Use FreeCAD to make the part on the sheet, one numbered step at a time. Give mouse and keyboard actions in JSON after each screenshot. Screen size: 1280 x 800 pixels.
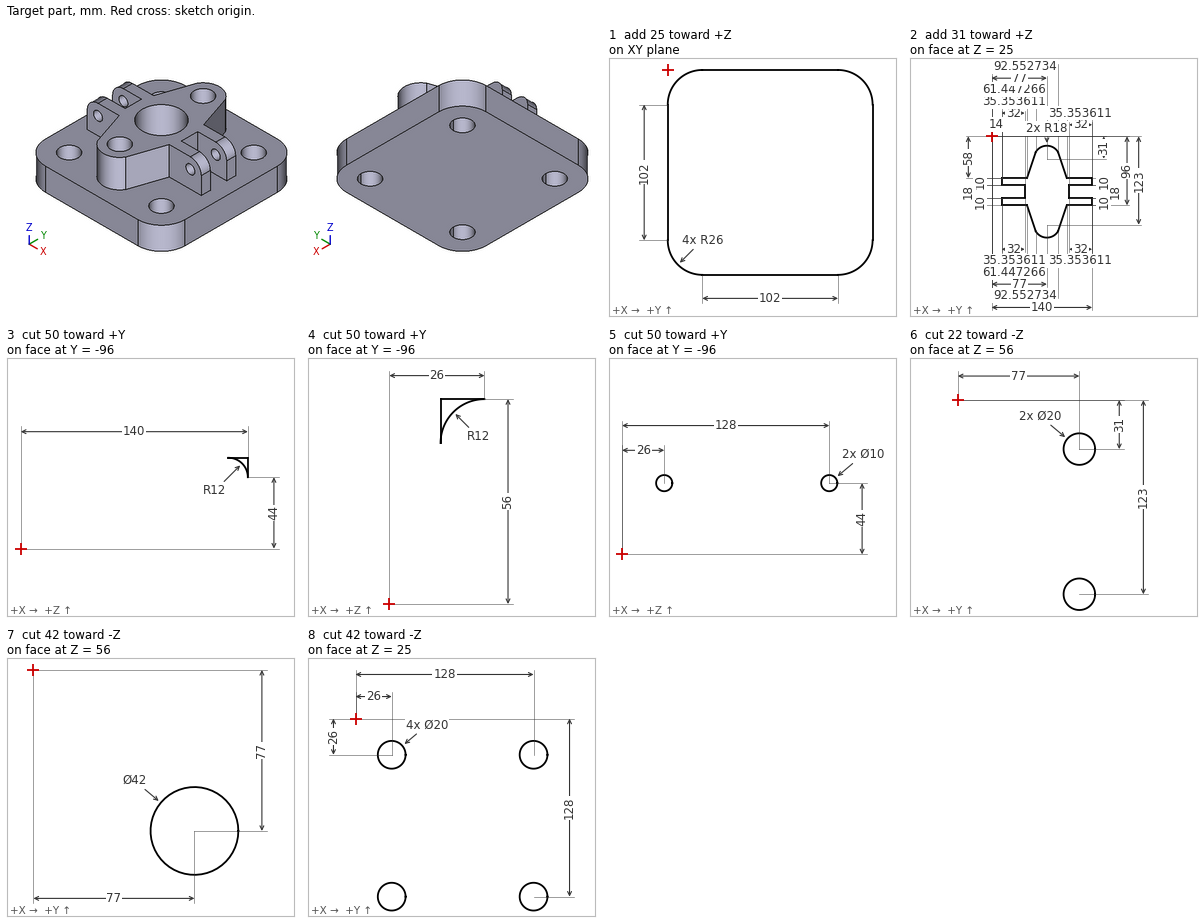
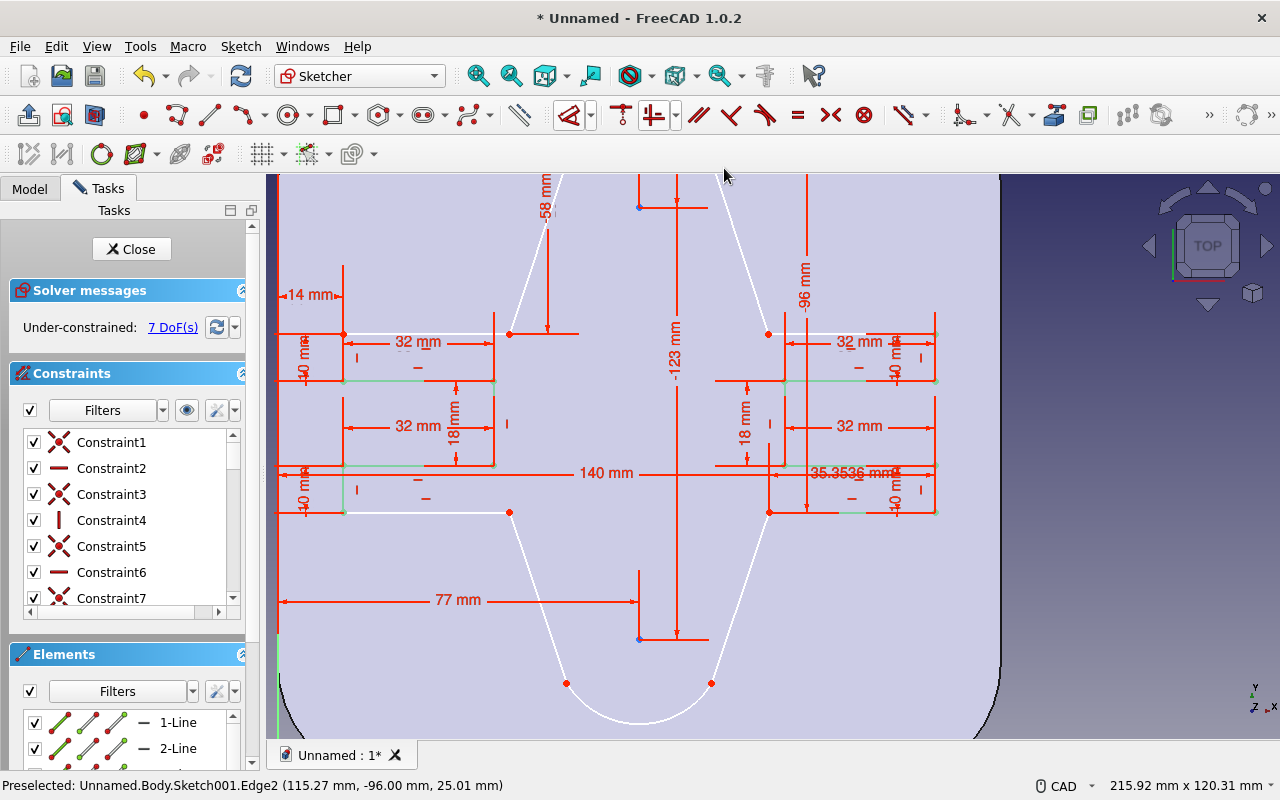
{"action": "left_click", "coordinate": [885, 334]}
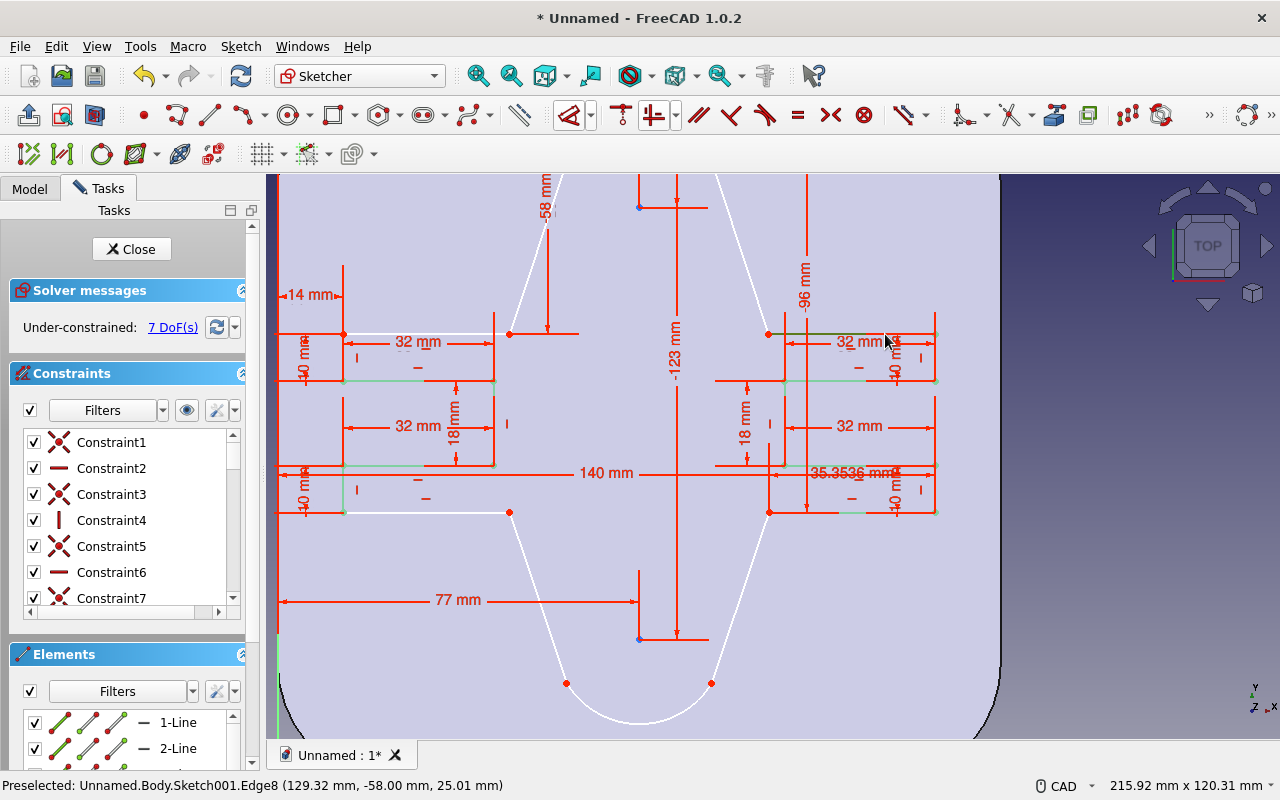
{"action": "key", "text": "l"}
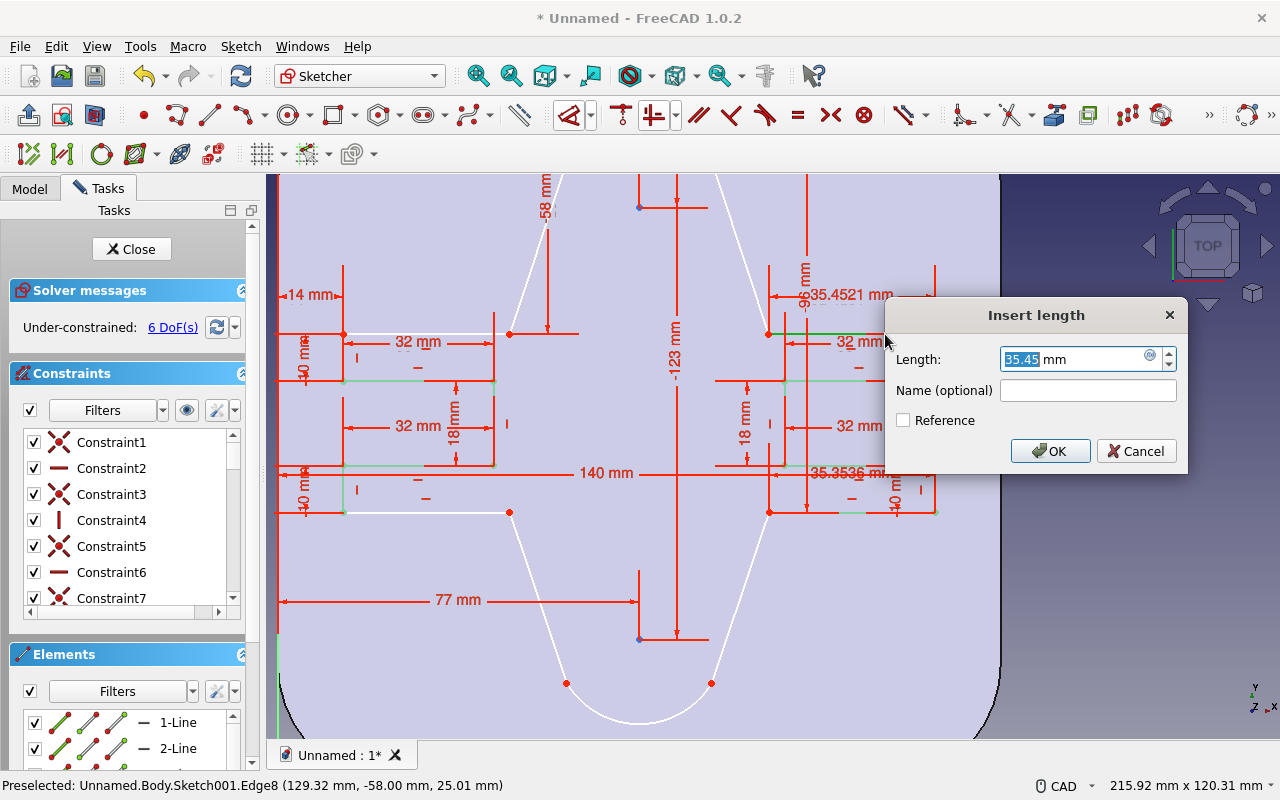
{"action": "type", "text": "35.353611"}
{"action": "key", "text": "Return"}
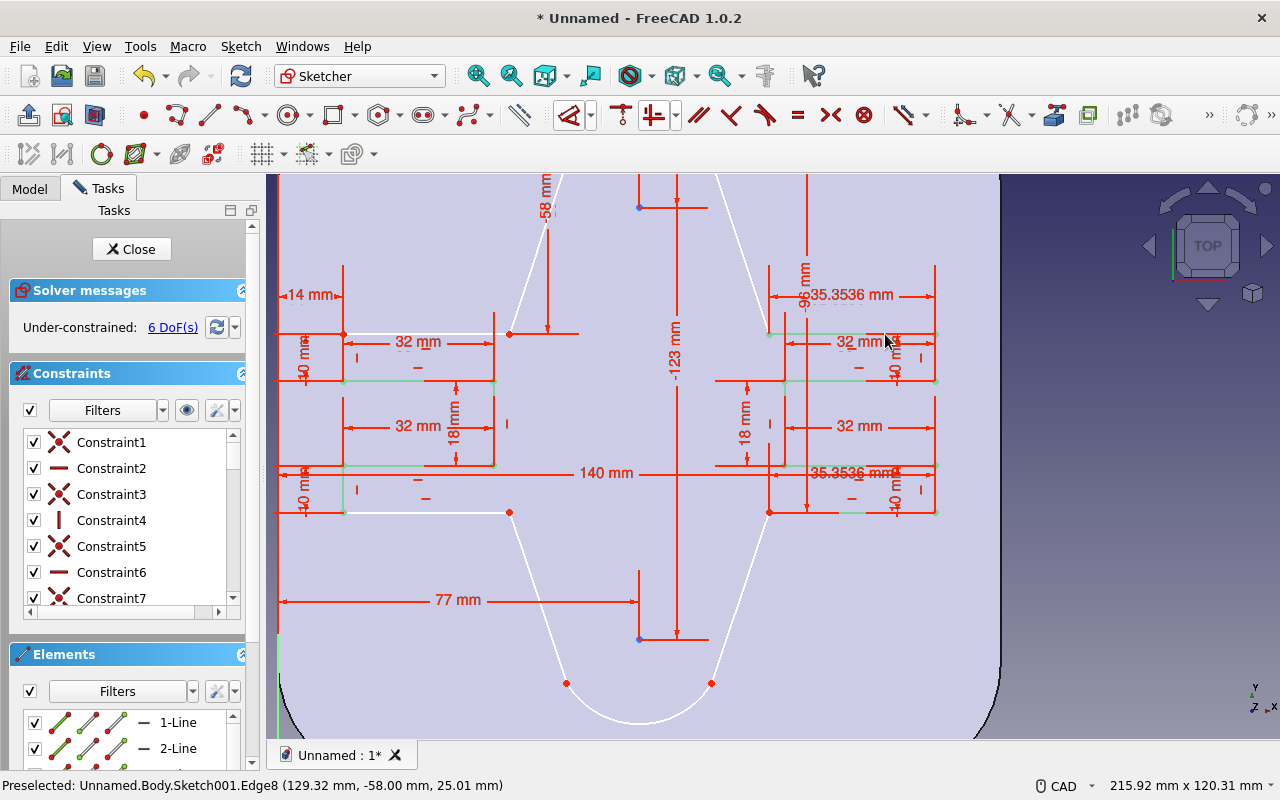
{"action": "left_click", "coordinate": [460, 334]}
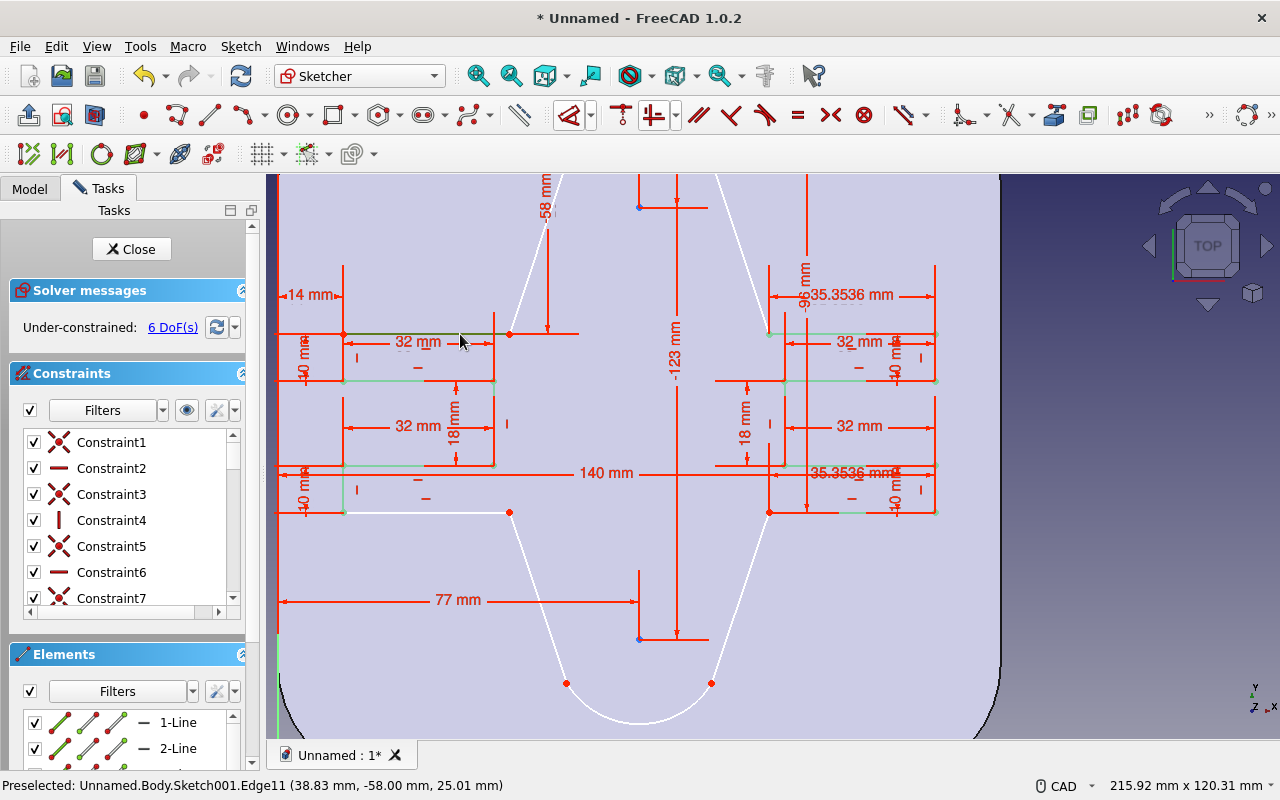
{"action": "key", "text": "l"}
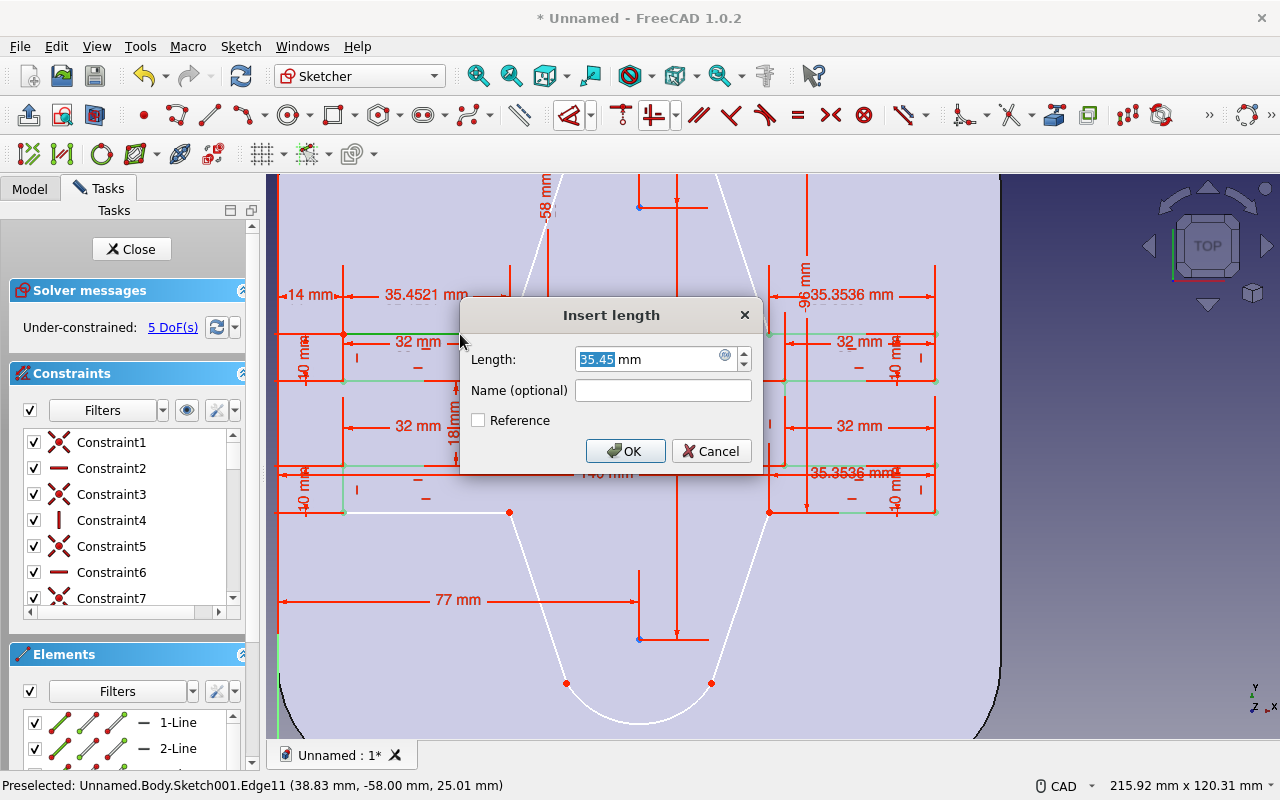
{"action": "type", "text": "35.353611"}
{"action": "key", "text": "Return"}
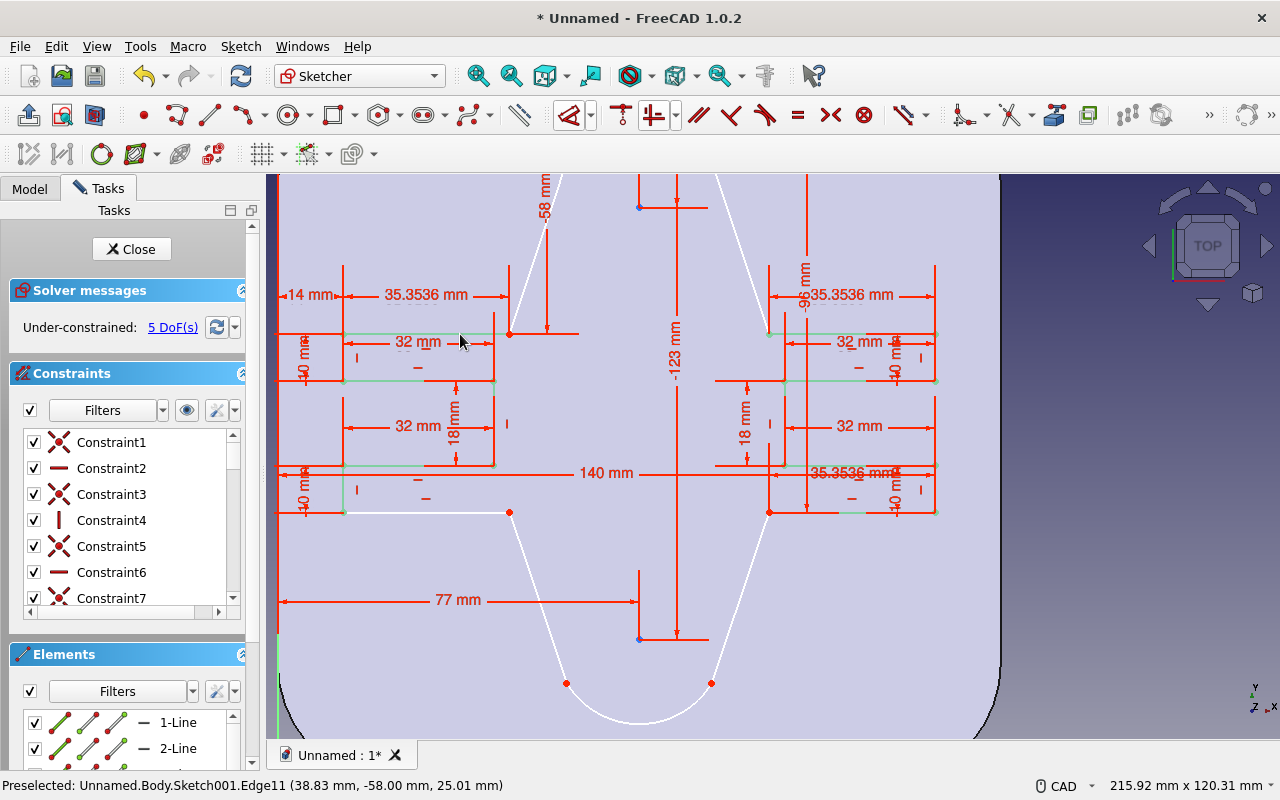
{"action": "left_click", "coordinate": [393, 513]}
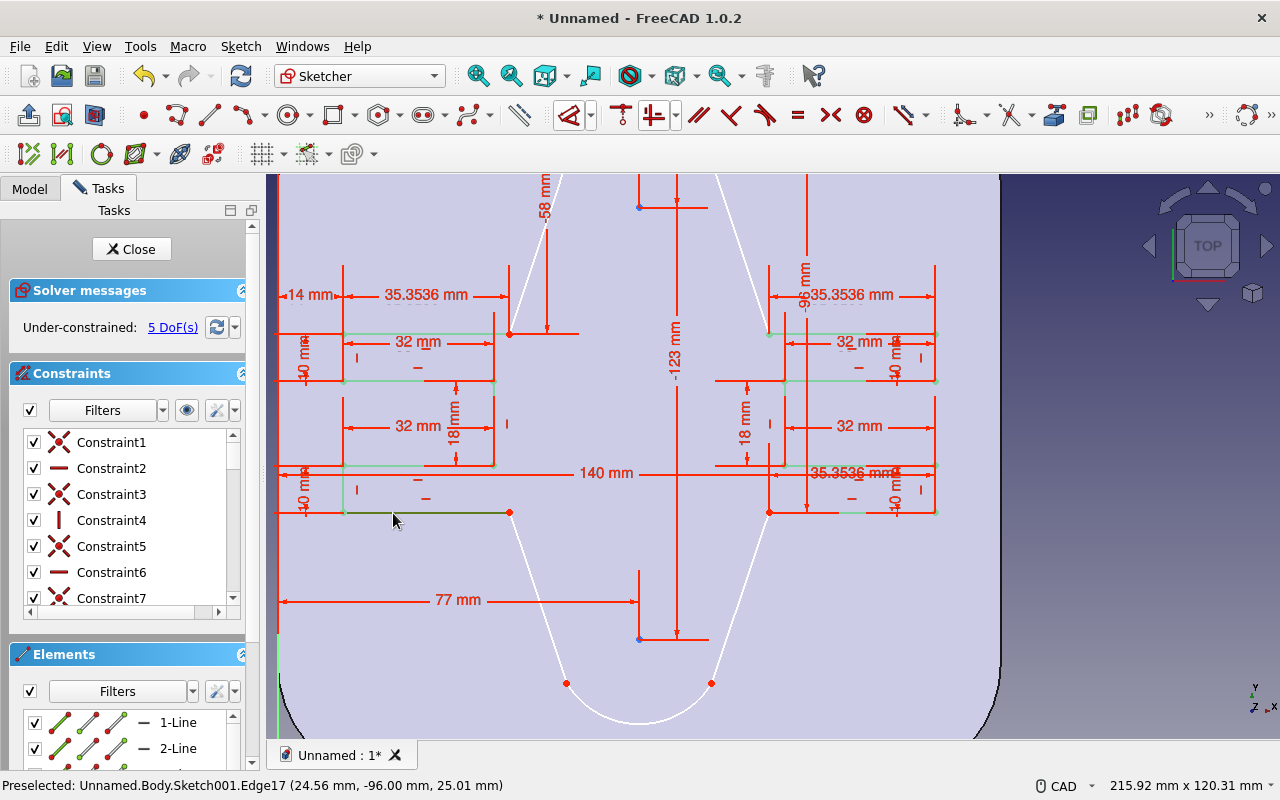
{"action": "left_click", "coordinate": [590, 116]}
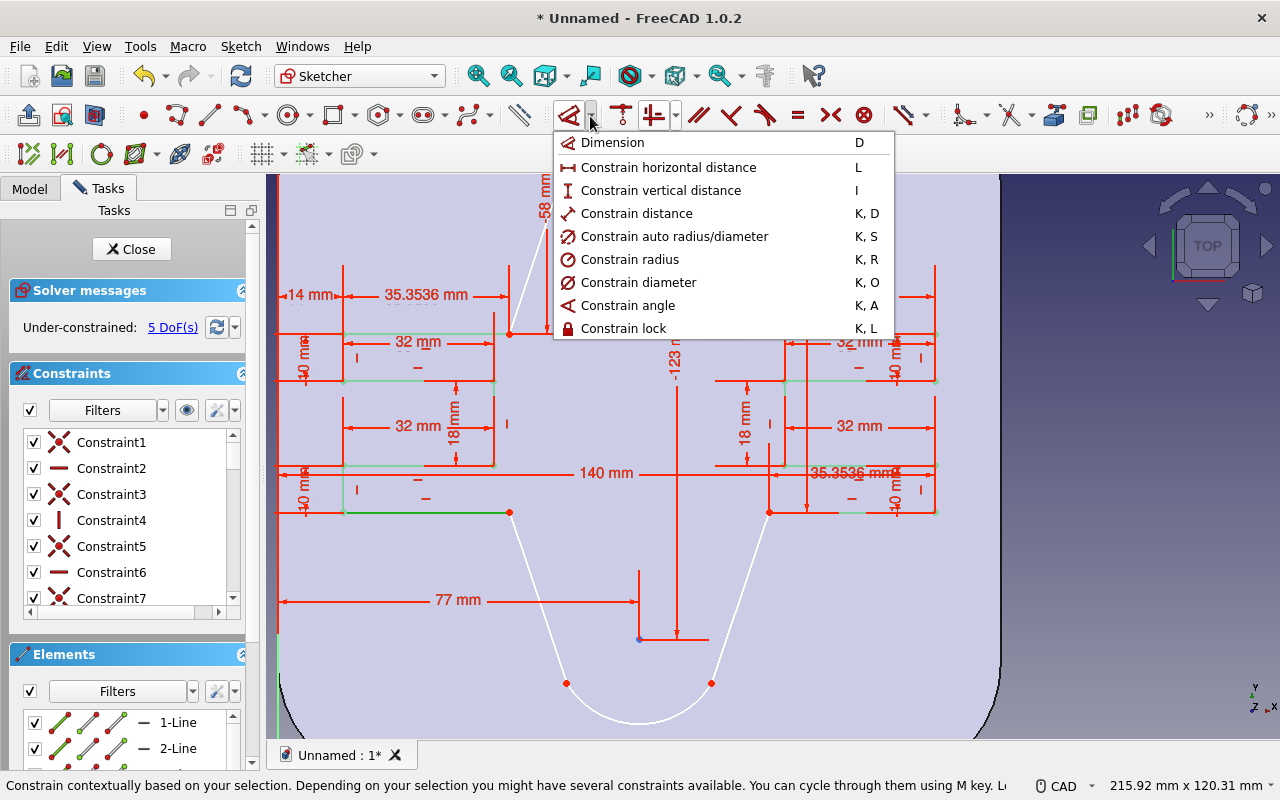
{"action": "left_click", "coordinate": [724, 168]}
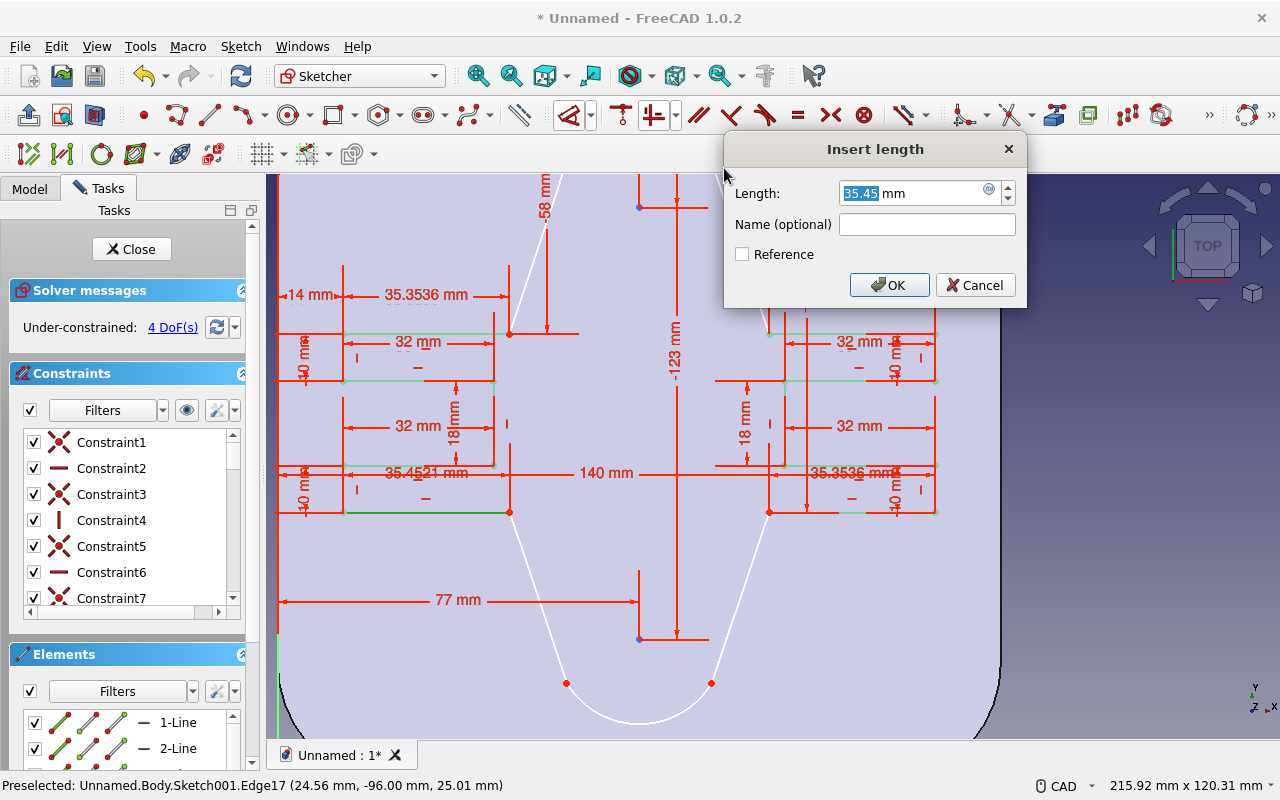
{"action": "type", "text": "35.353611"}
{"action": "key", "text": "Return"}